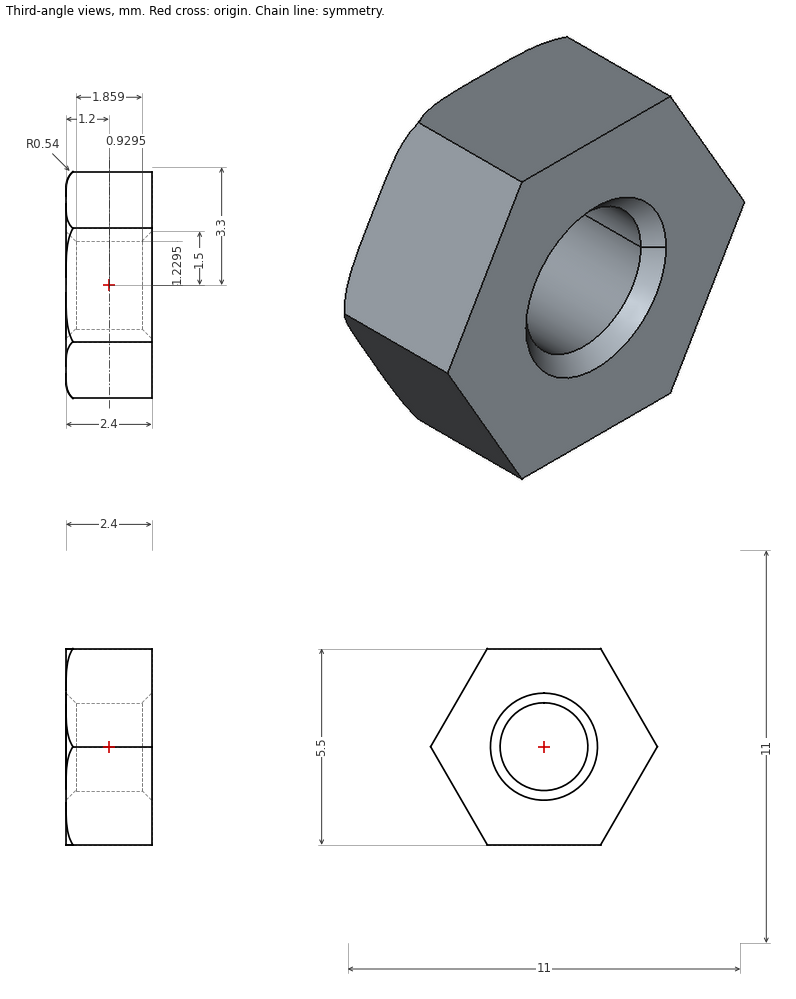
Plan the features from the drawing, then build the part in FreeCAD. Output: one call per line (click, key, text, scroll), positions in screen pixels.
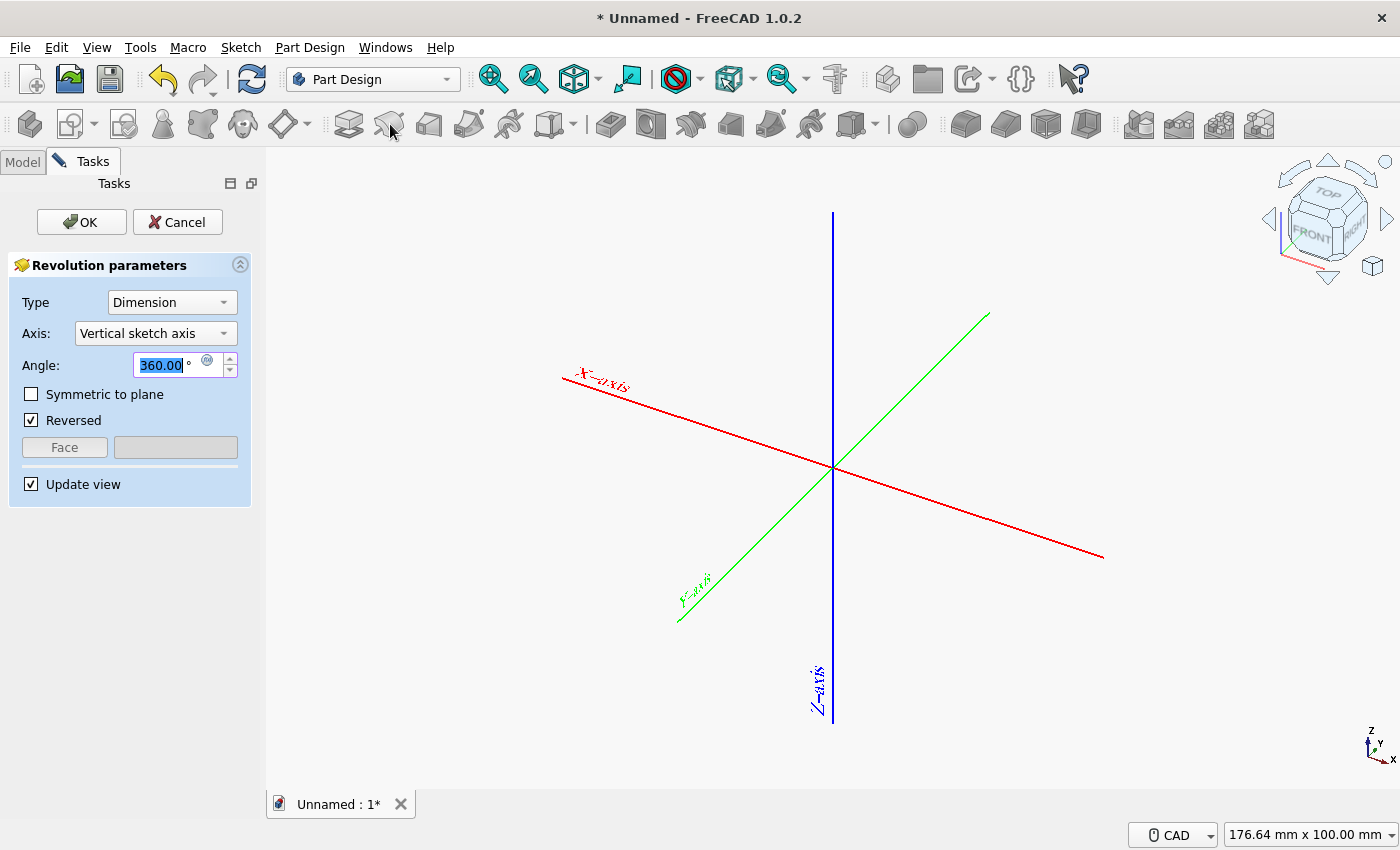
click(156, 334)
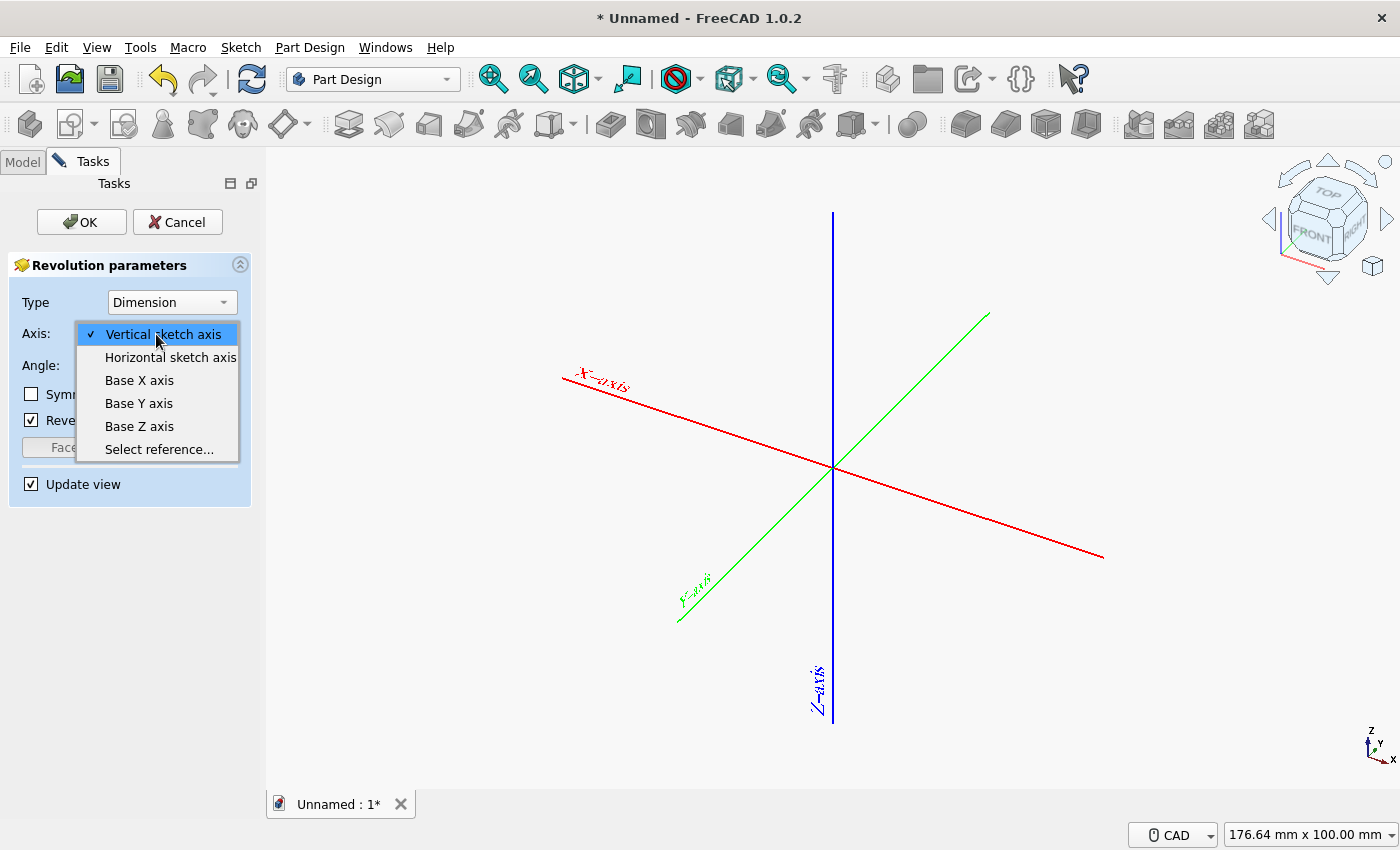
click(156, 358)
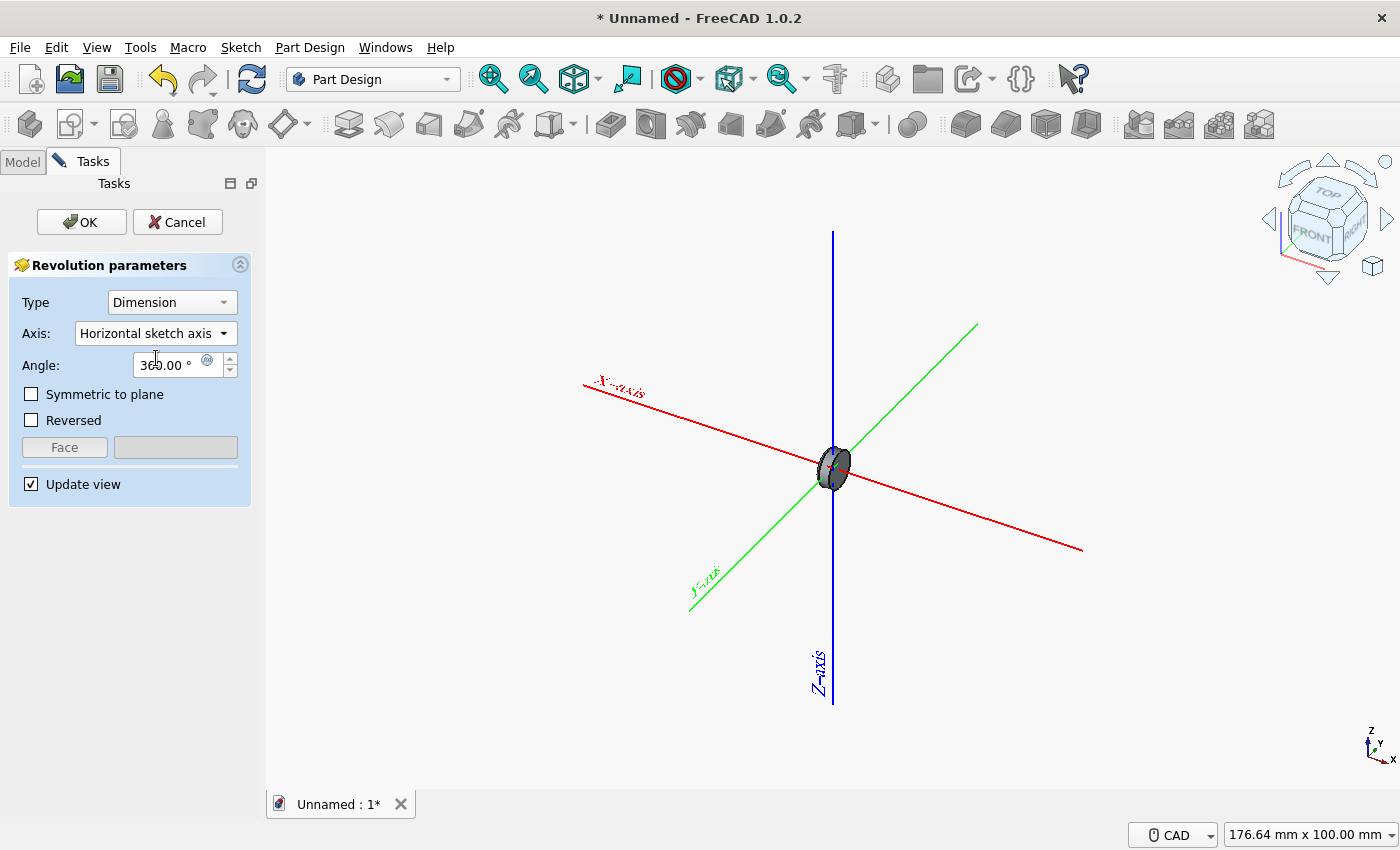
click(82, 222)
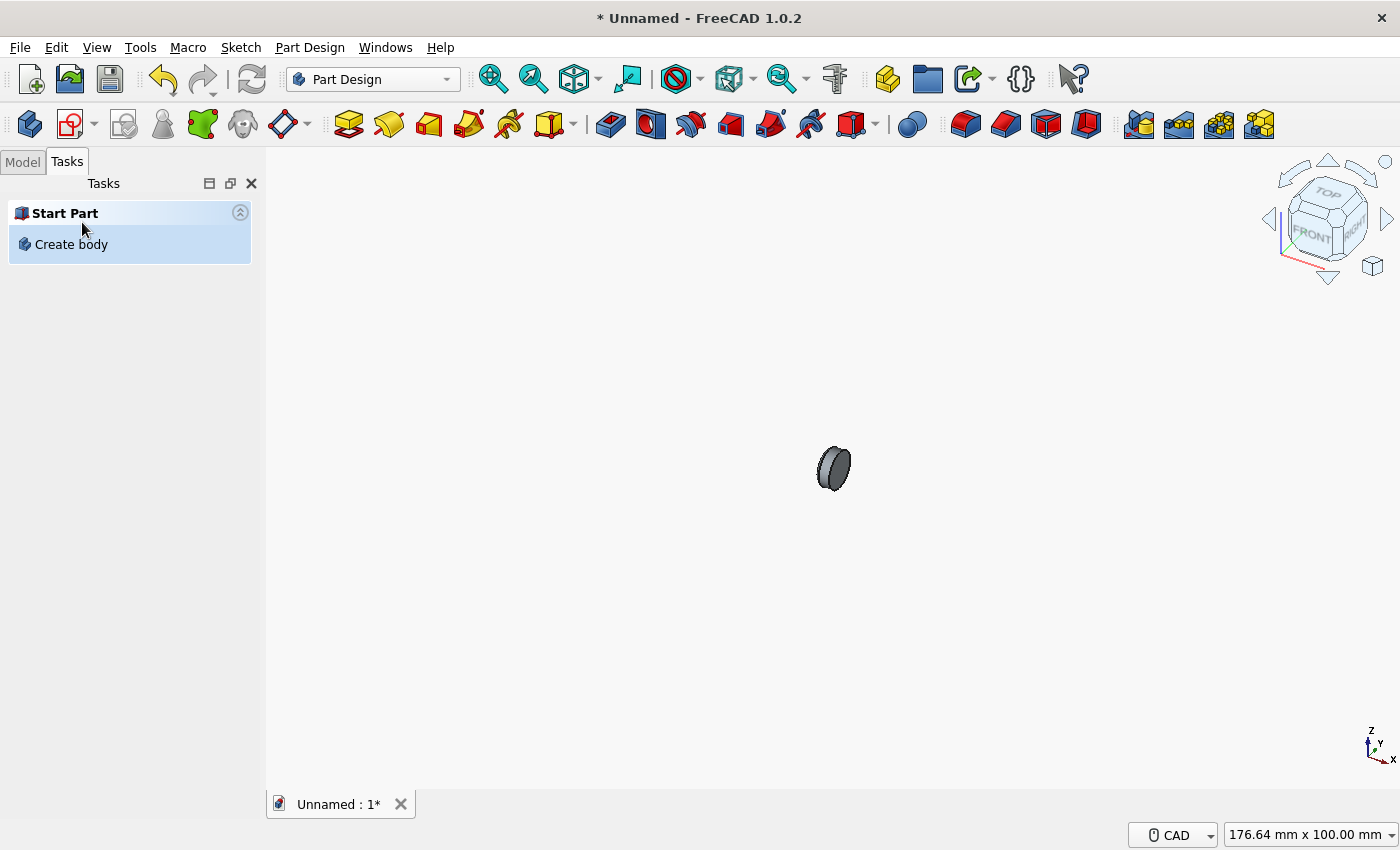
click(494, 80)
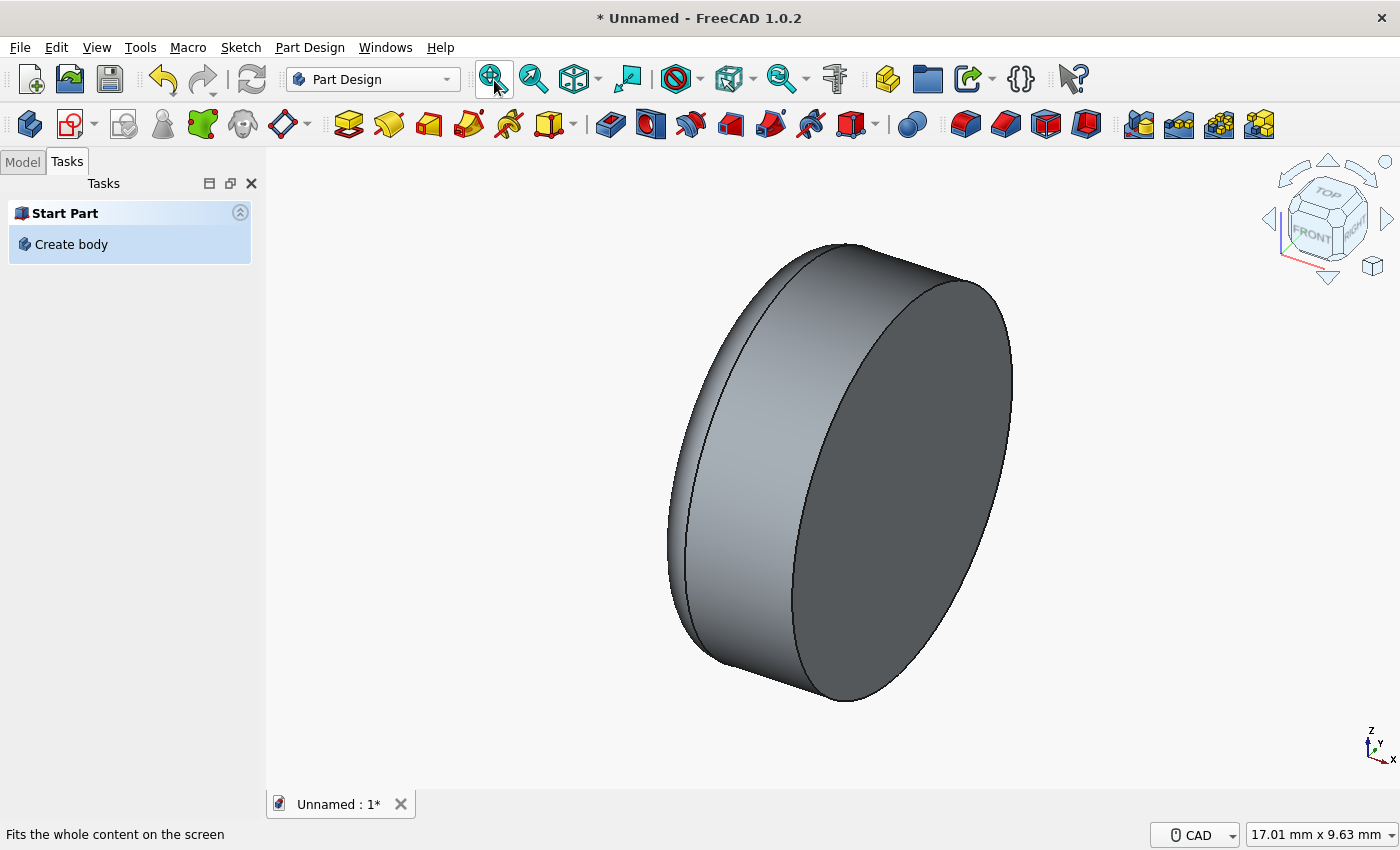
click(70, 124)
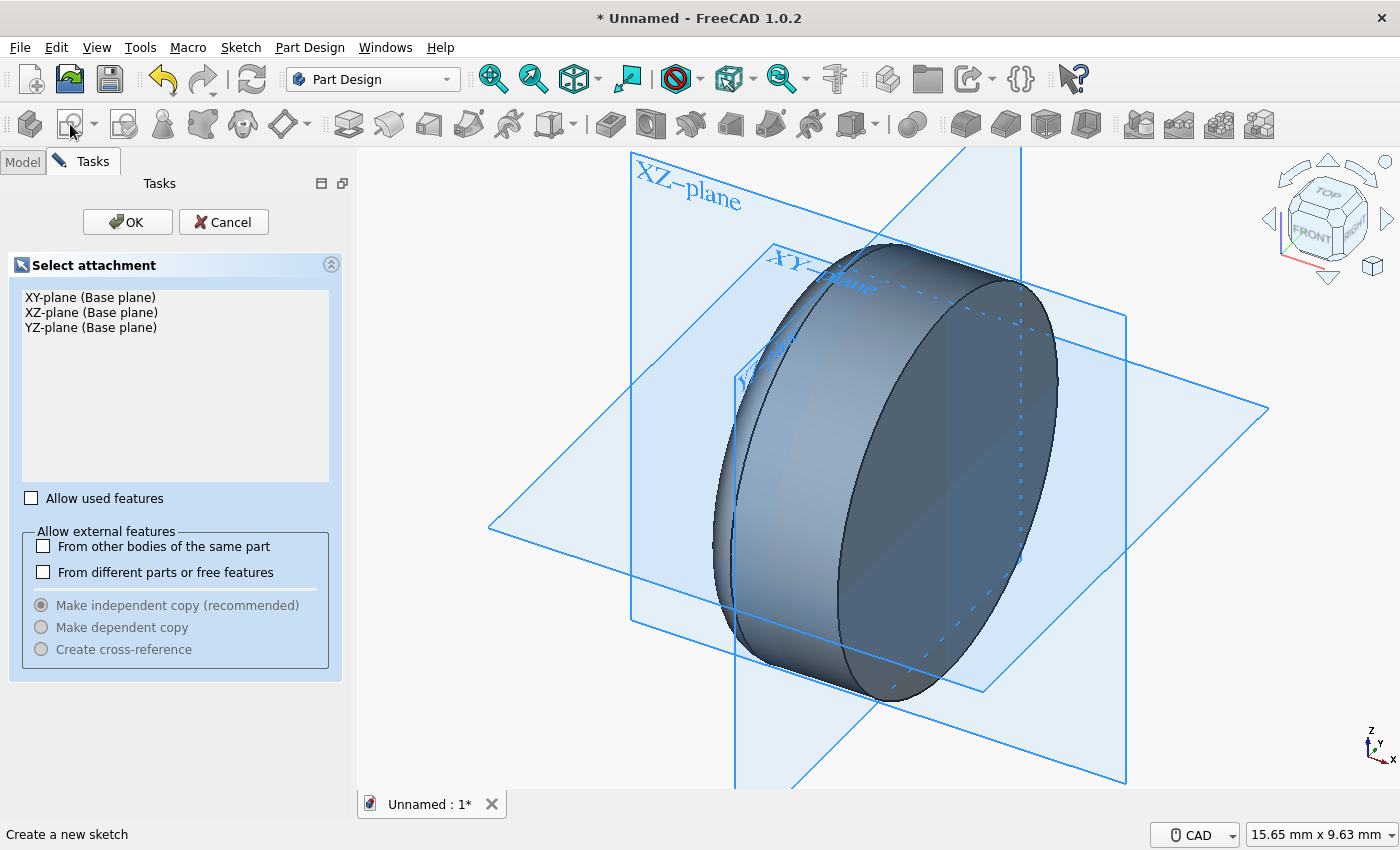
click(82, 298)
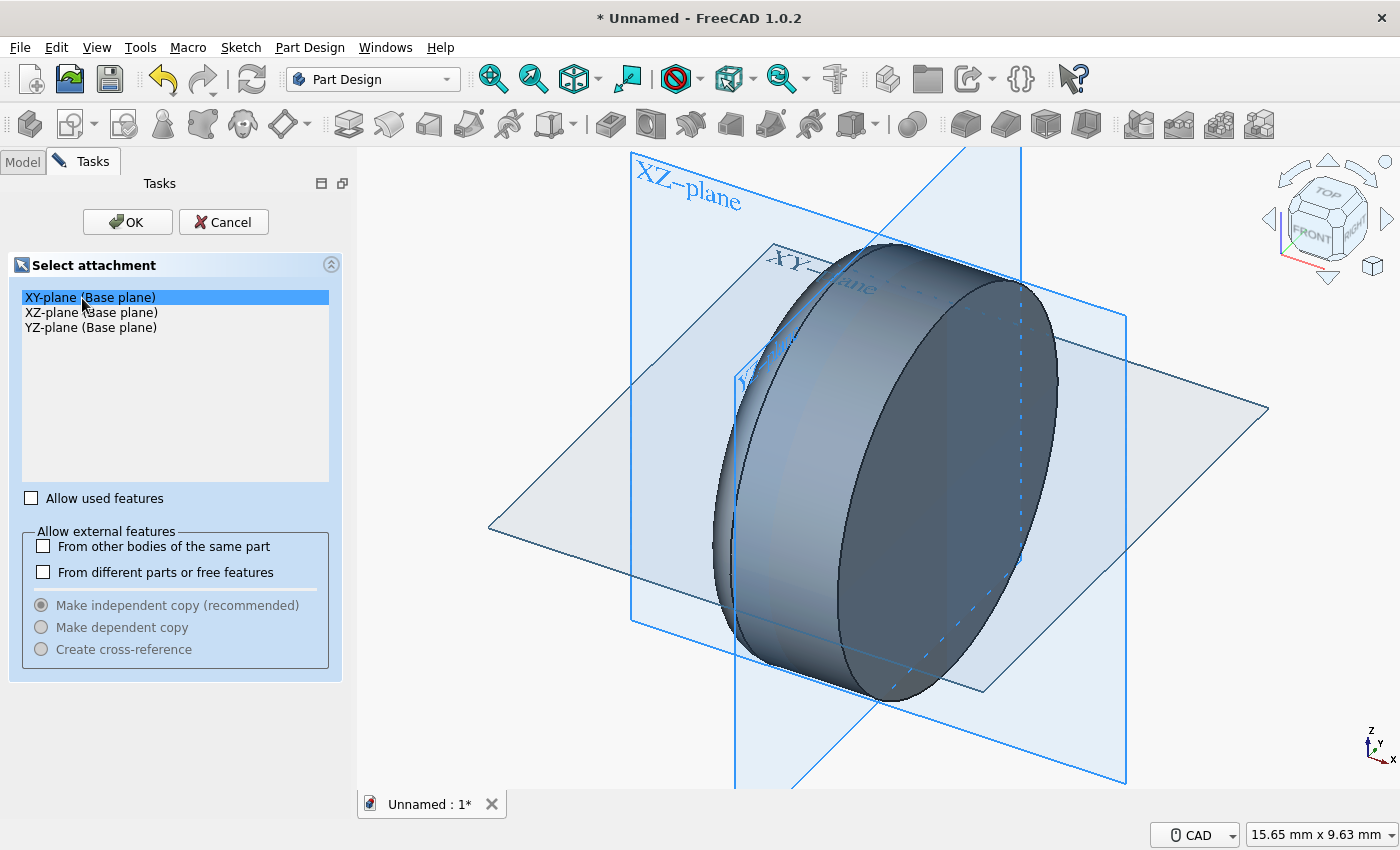
click(128, 222)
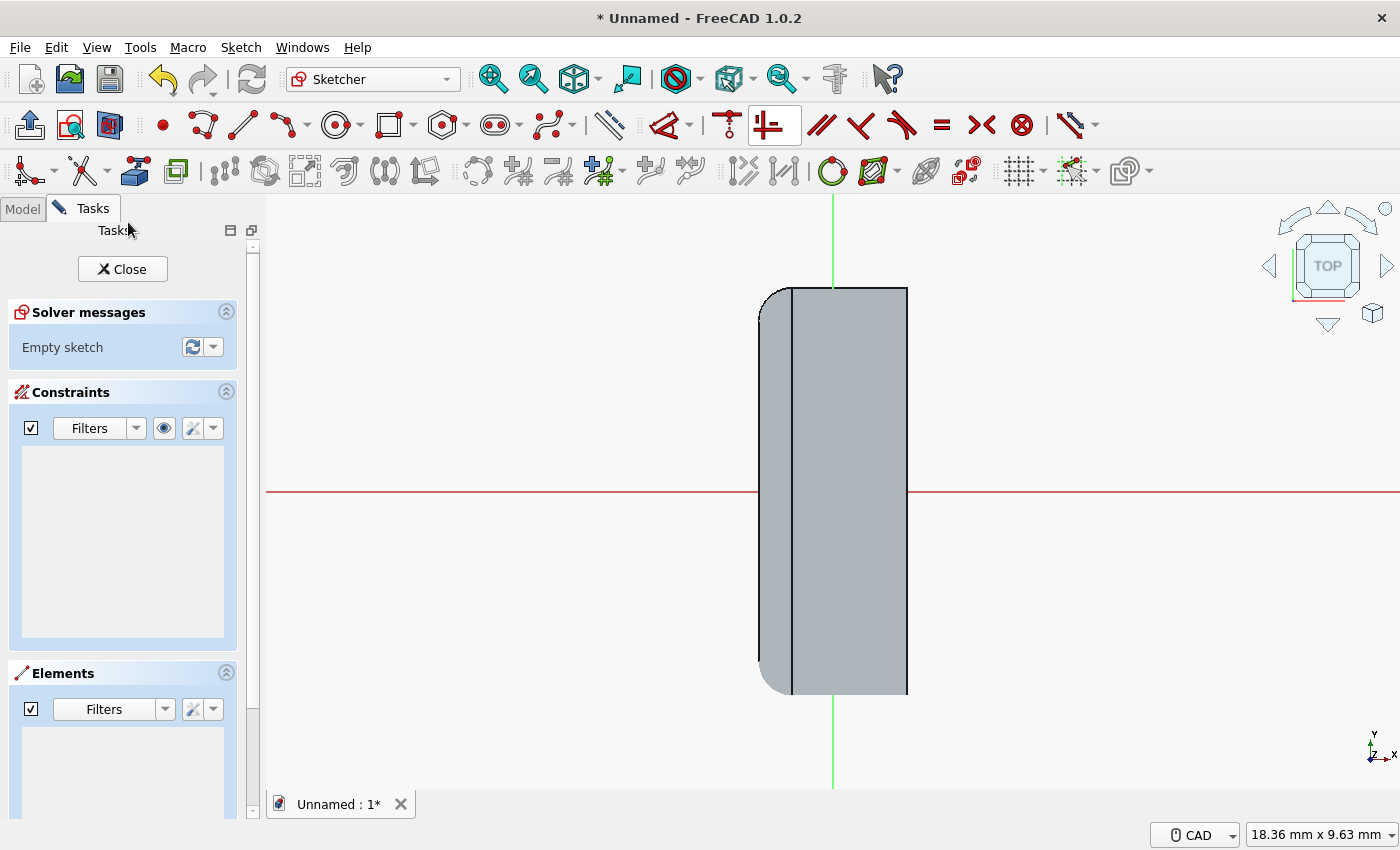
click(110, 126)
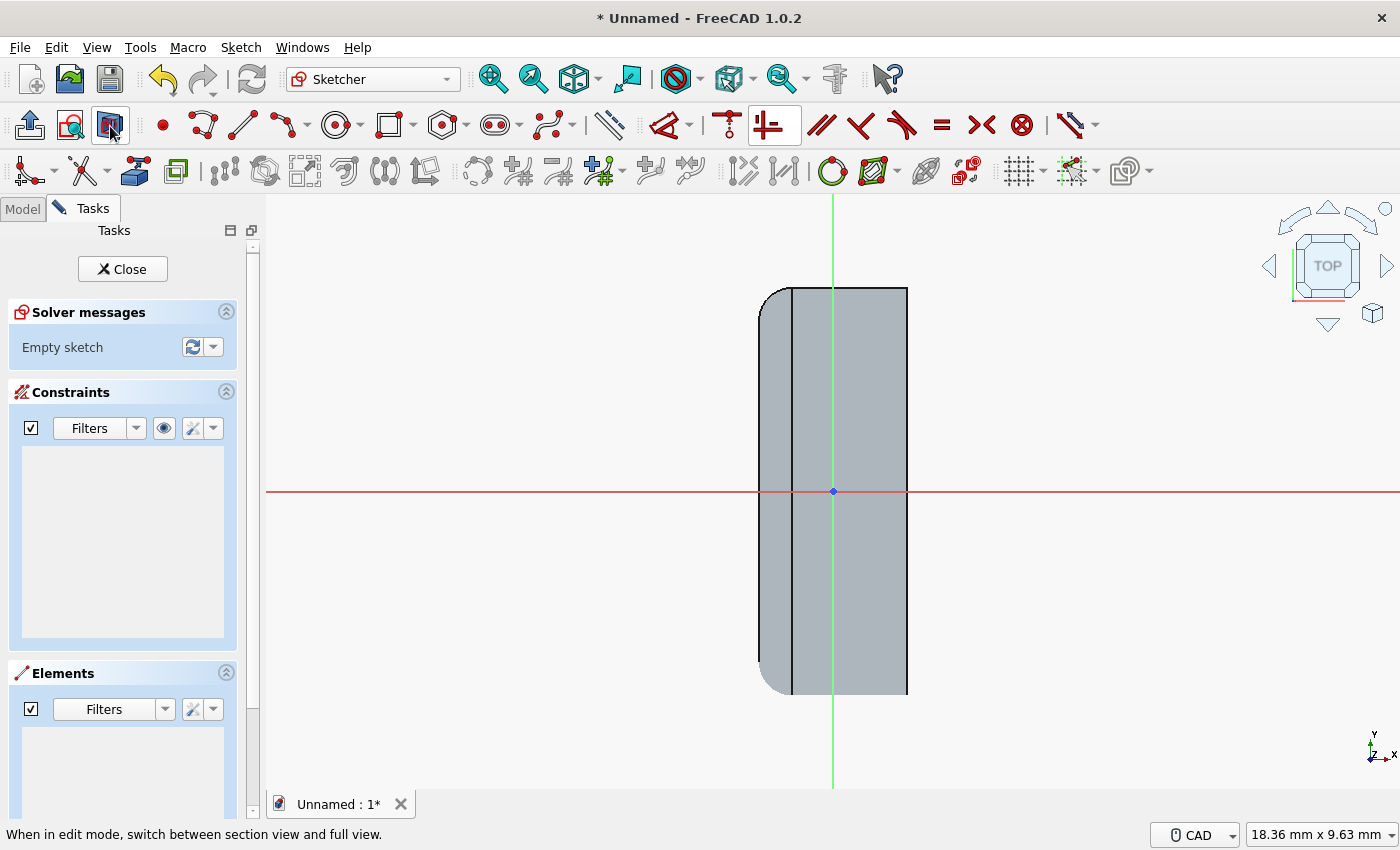
scroll(855, 430, up, 7)